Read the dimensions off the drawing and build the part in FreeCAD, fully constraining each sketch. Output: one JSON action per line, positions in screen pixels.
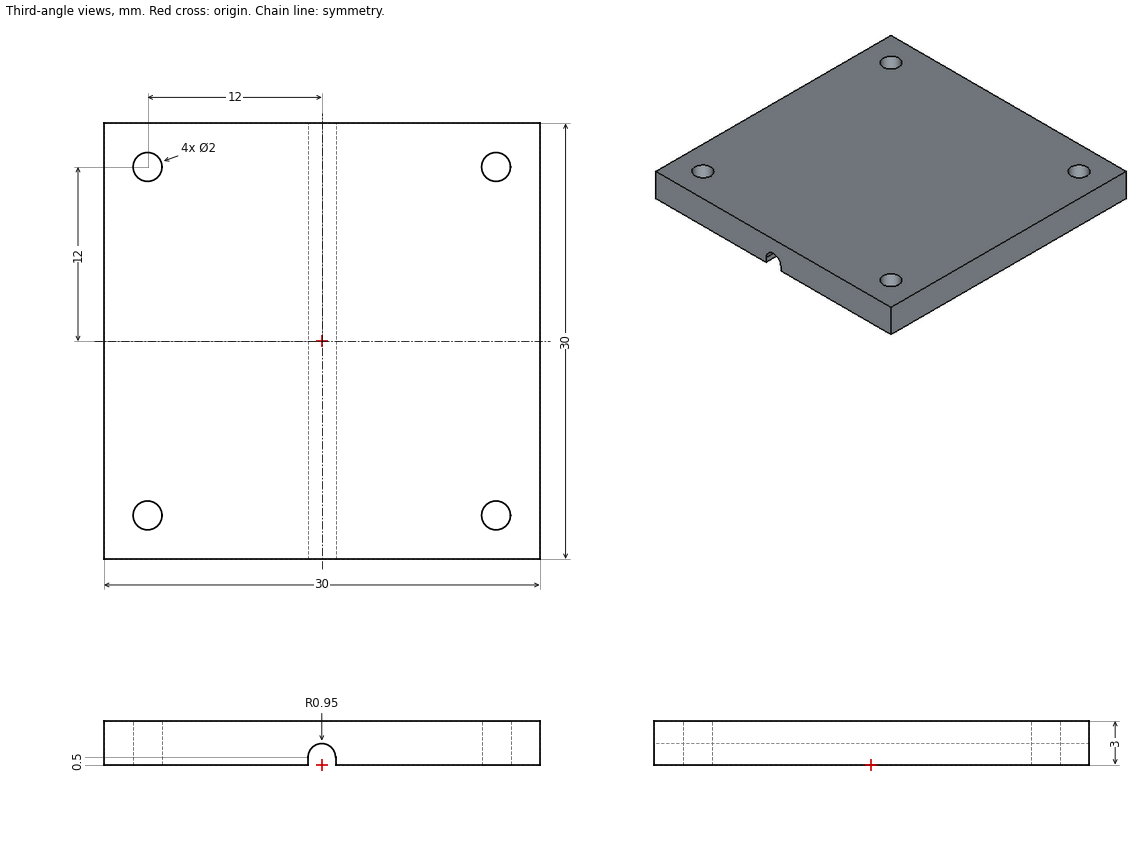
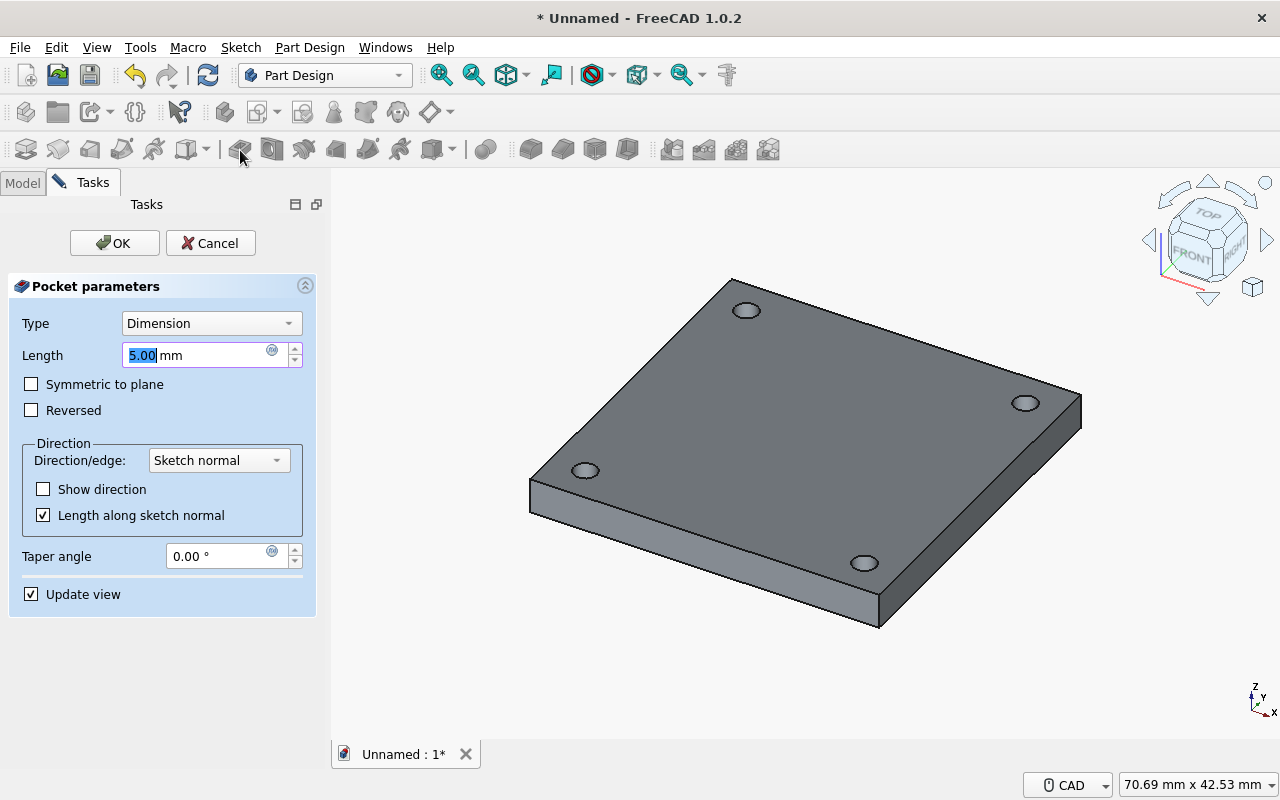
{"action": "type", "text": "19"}
{"action": "key", "text": "Tab"}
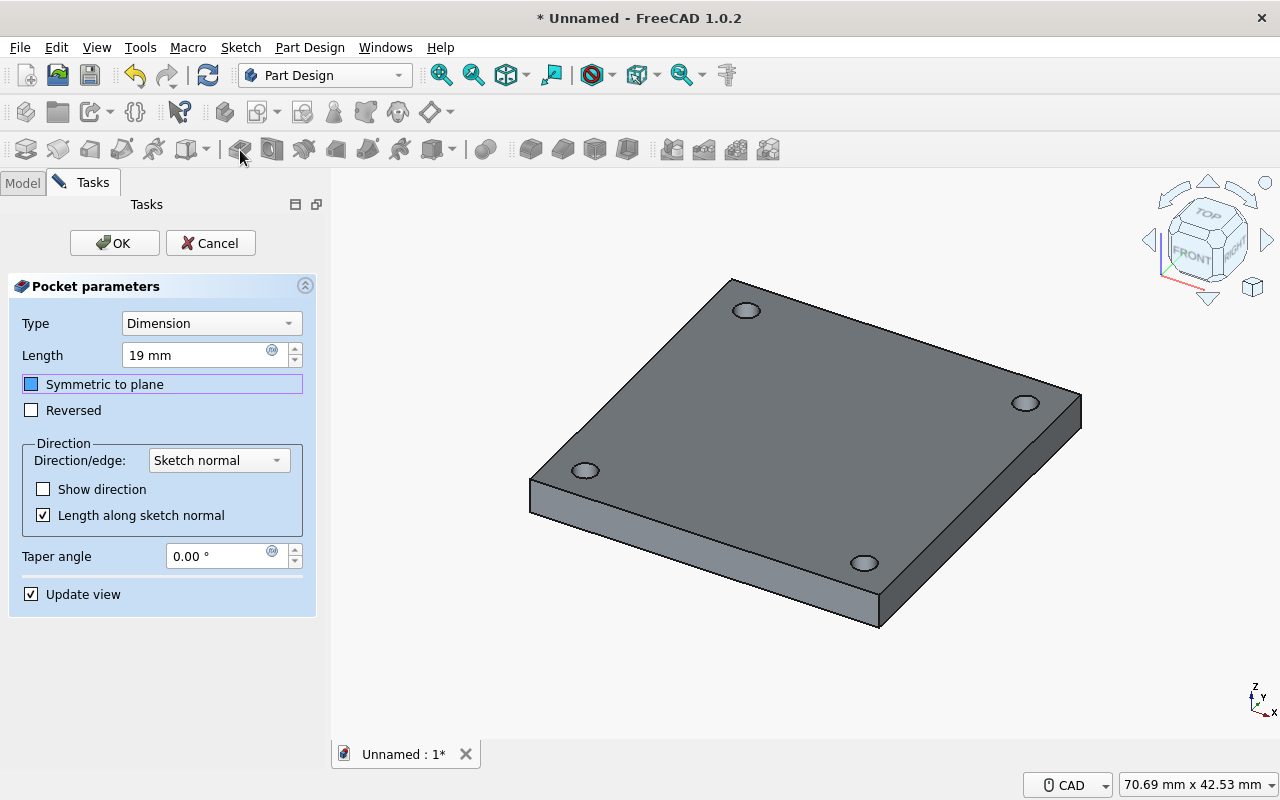
{"action": "left_click", "coordinate": [115, 243]}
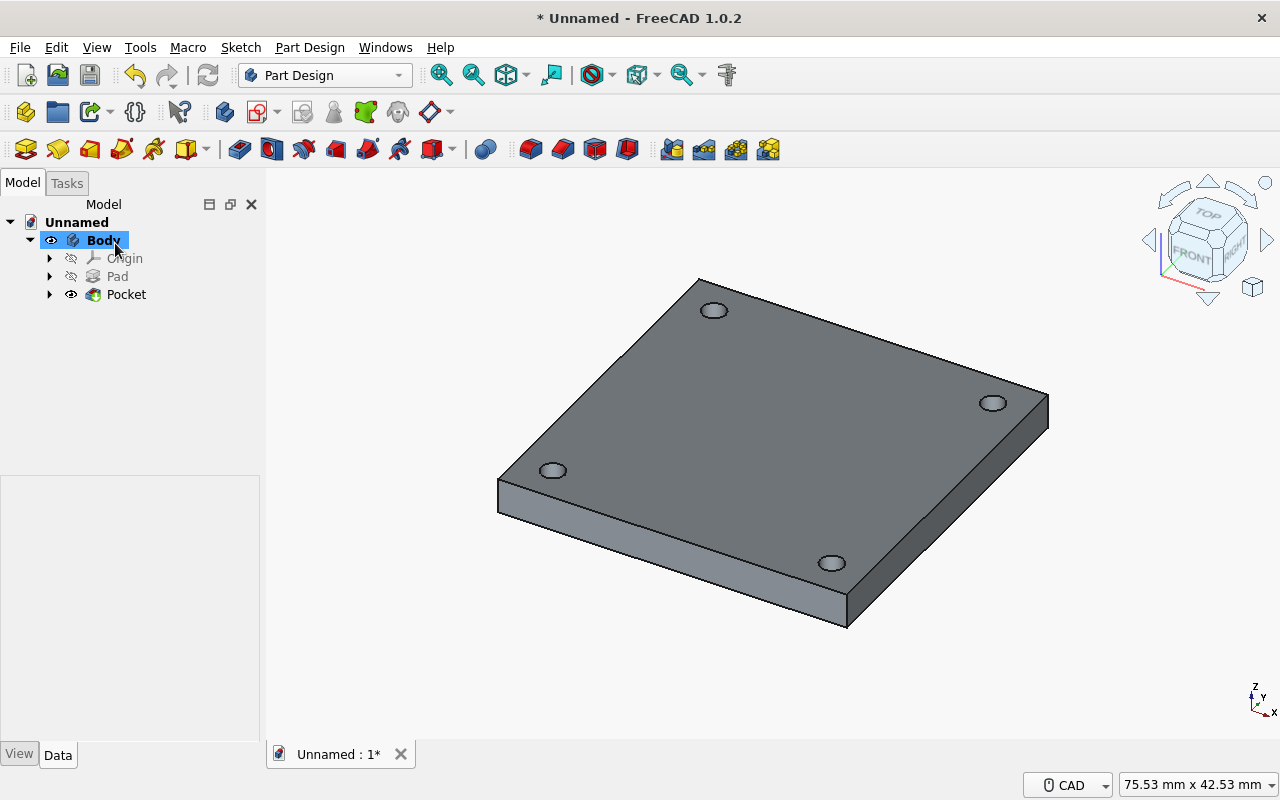
{"action": "left_click", "coordinate": [822, 602]}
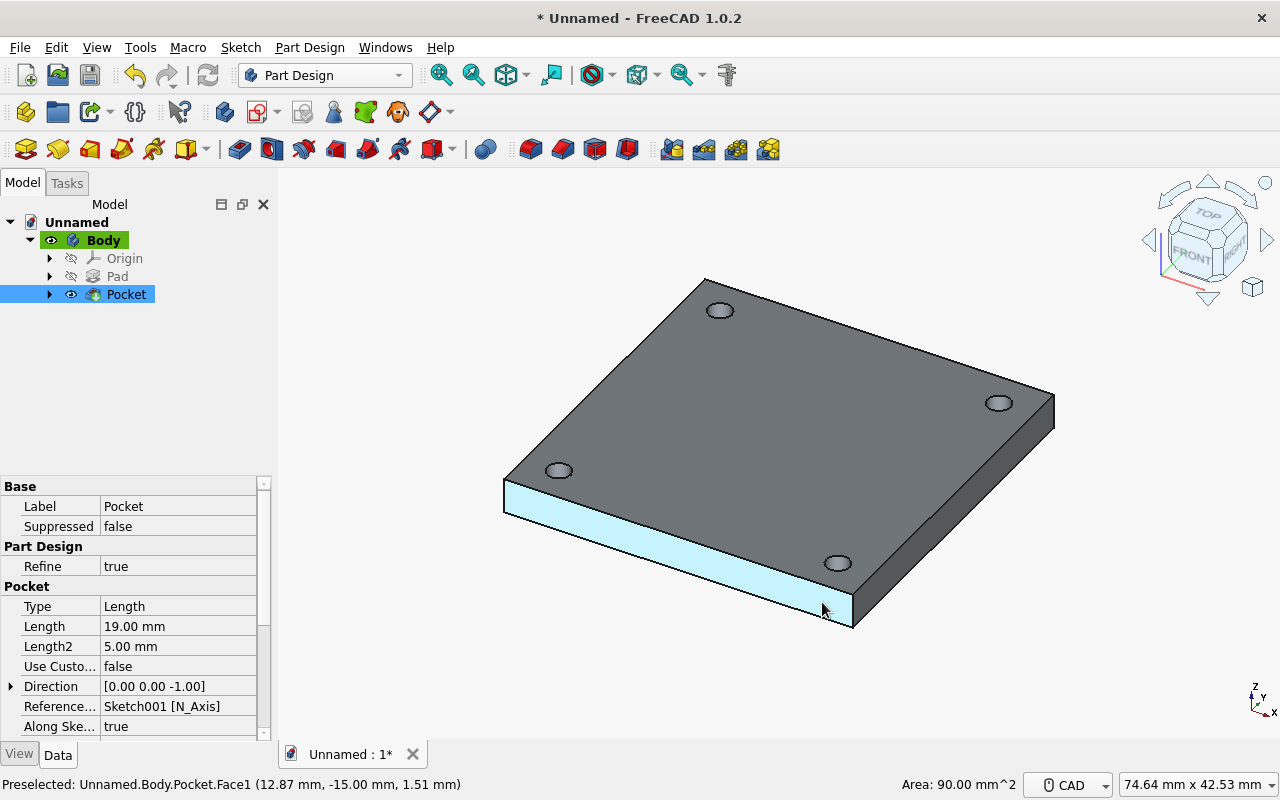
{"action": "left_click", "coordinate": [258, 112]}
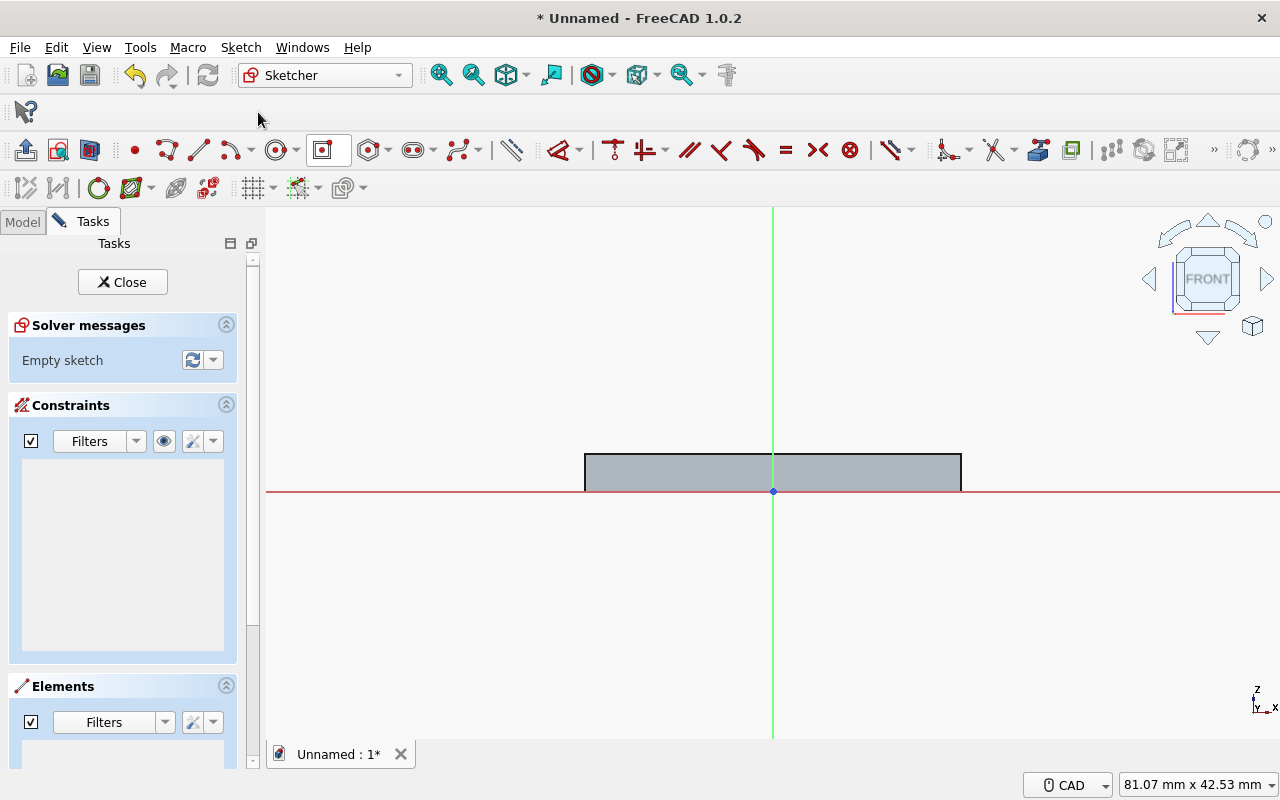
{"action": "scroll", "coordinate": [777, 483], "scroll_direction": "up", "scroll_amount": 15}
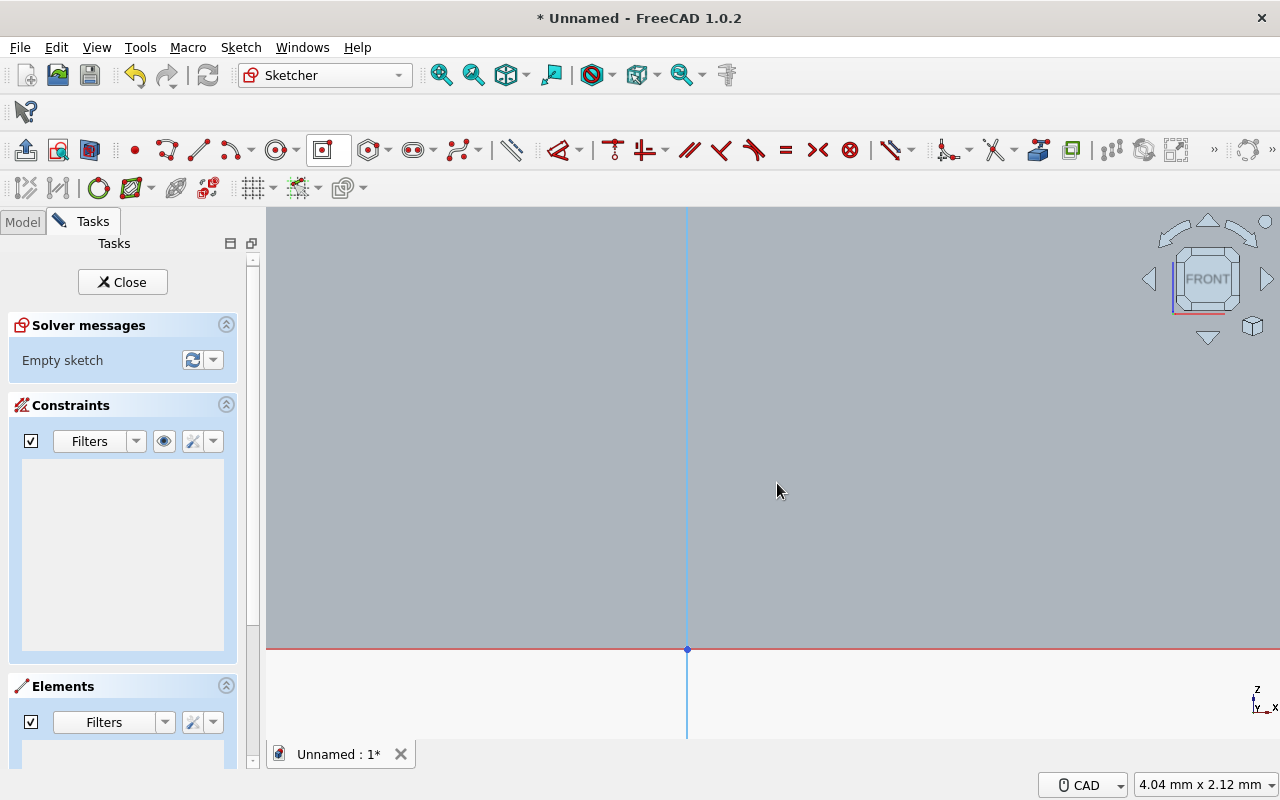
{"action": "left_click", "coordinate": [168, 150]}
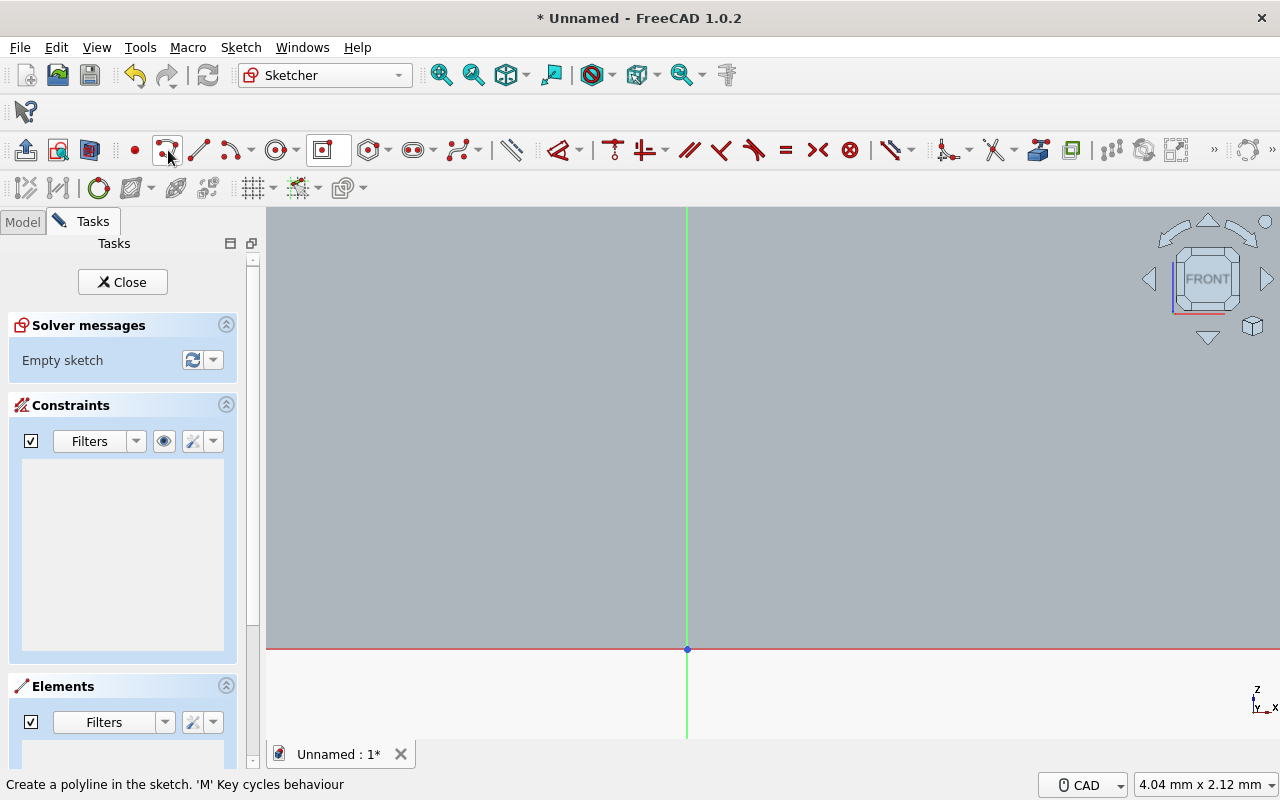
{"action": "left_click", "coordinate": [448, 523]}
{"action": "left_click", "coordinate": [448, 649]}
{"action": "left_click", "coordinate": [926, 640]}
{"action": "left_click", "coordinate": [926, 523]}
{"action": "right_click", "coordinate": [926, 523]}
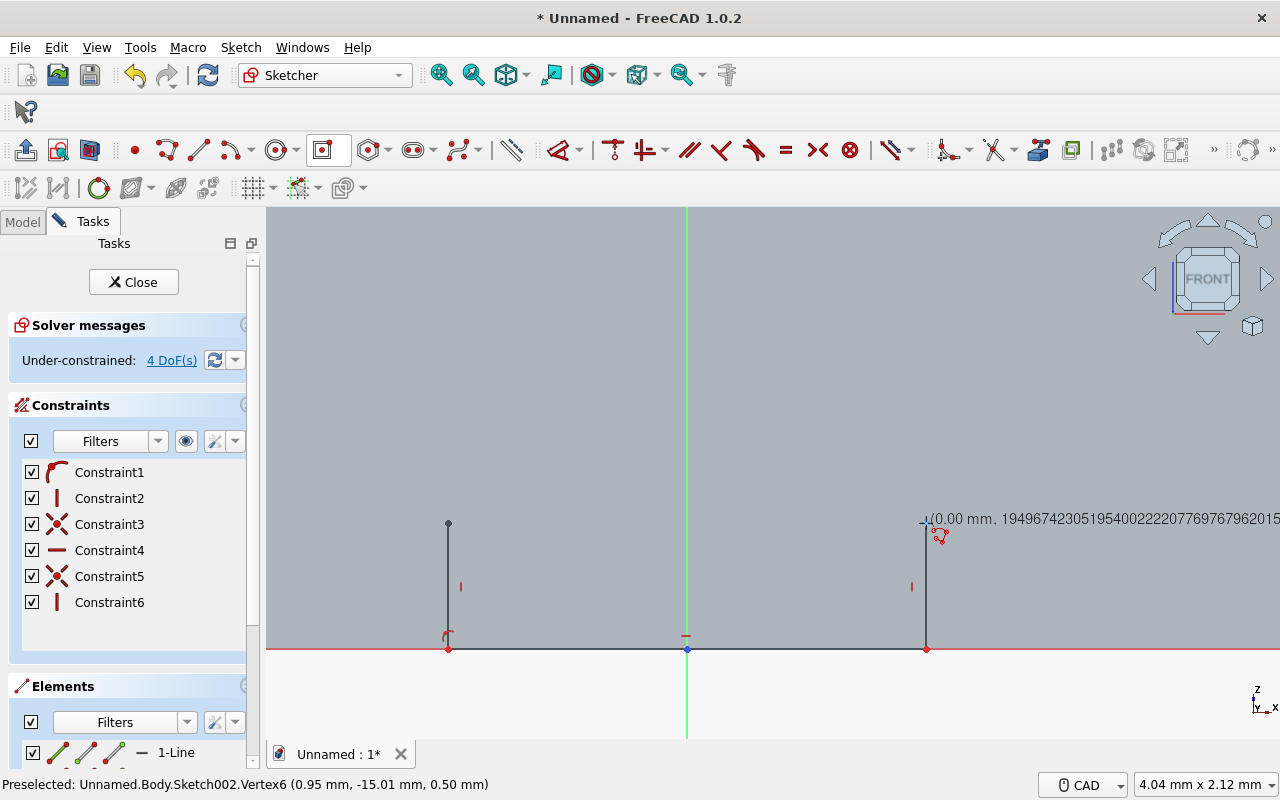
{"action": "key", "text": "g 3 a"}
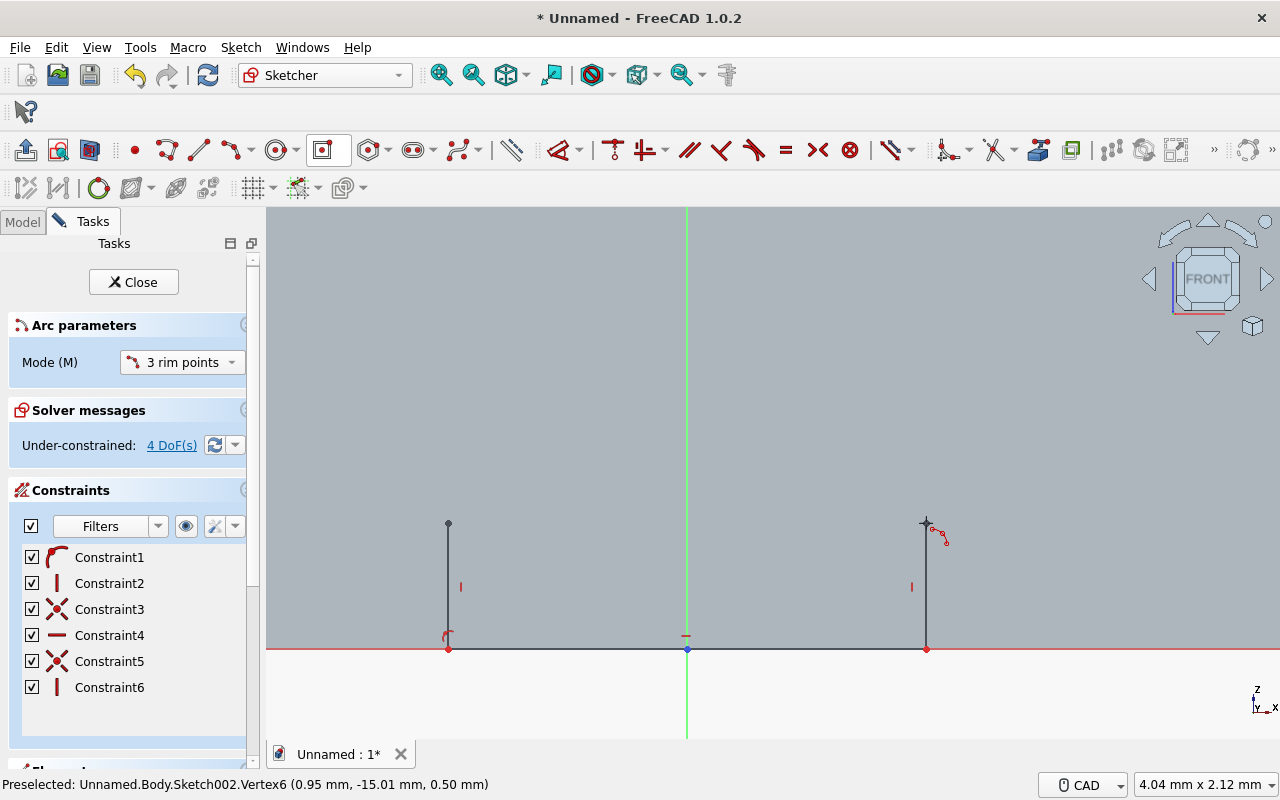
{"action": "left_click", "coordinate": [926, 524]}
{"action": "left_click", "coordinate": [448, 524]}
{"action": "left_click", "coordinate": [761, 296]}
{"action": "key", "text": "Escape"}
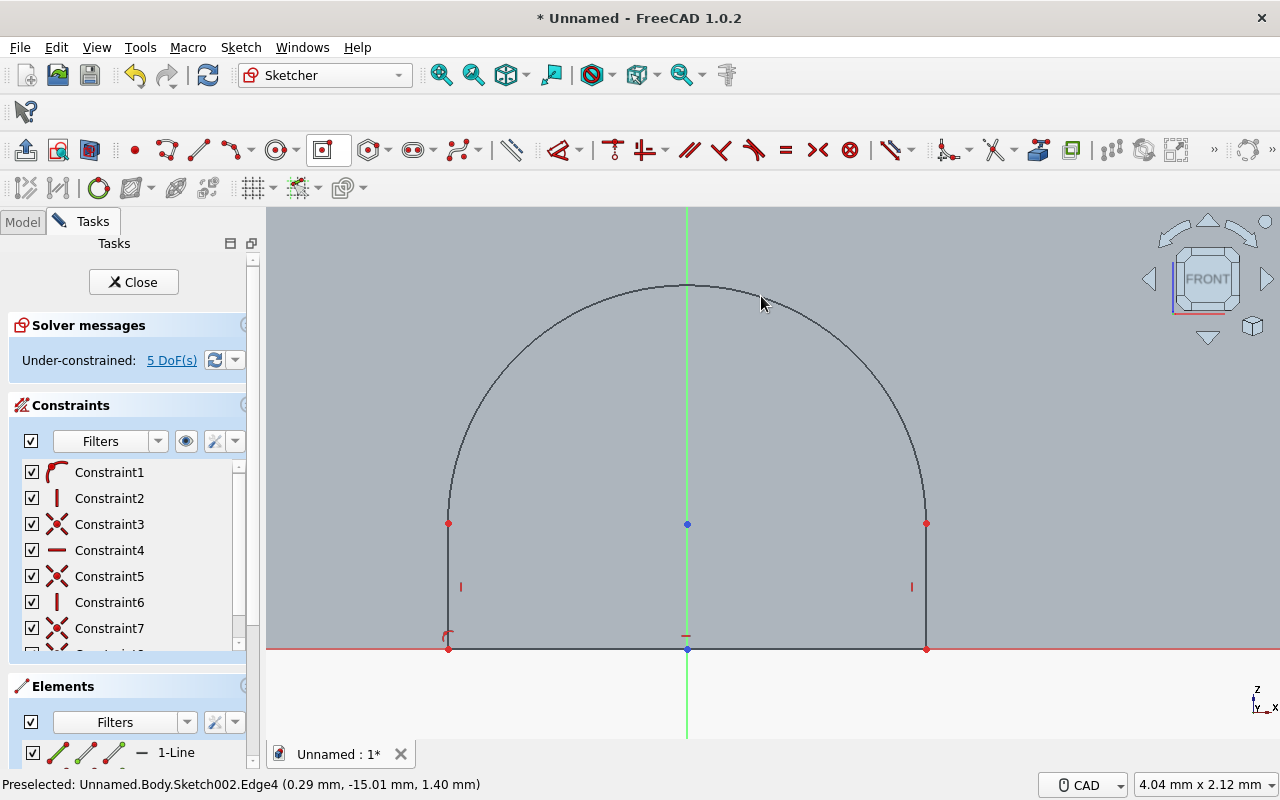
{"action": "left_click", "coordinate": [448, 562]}